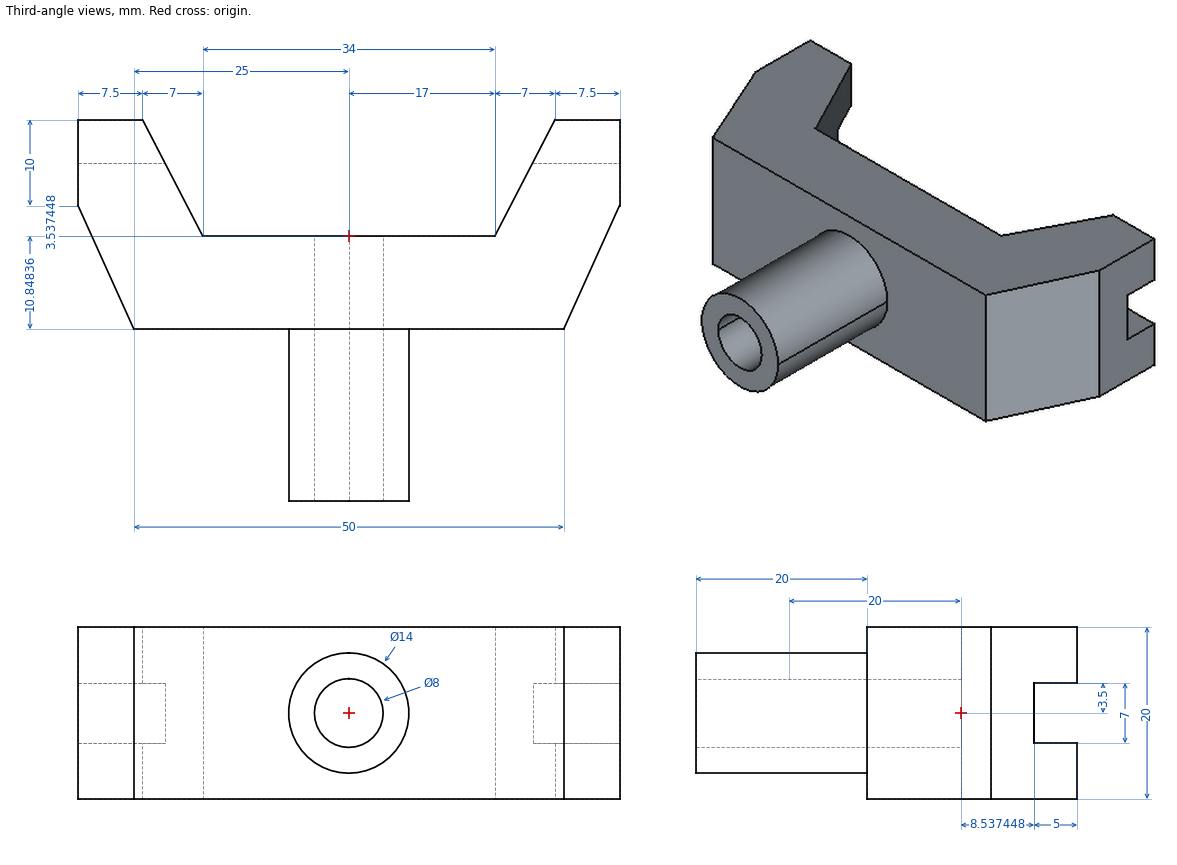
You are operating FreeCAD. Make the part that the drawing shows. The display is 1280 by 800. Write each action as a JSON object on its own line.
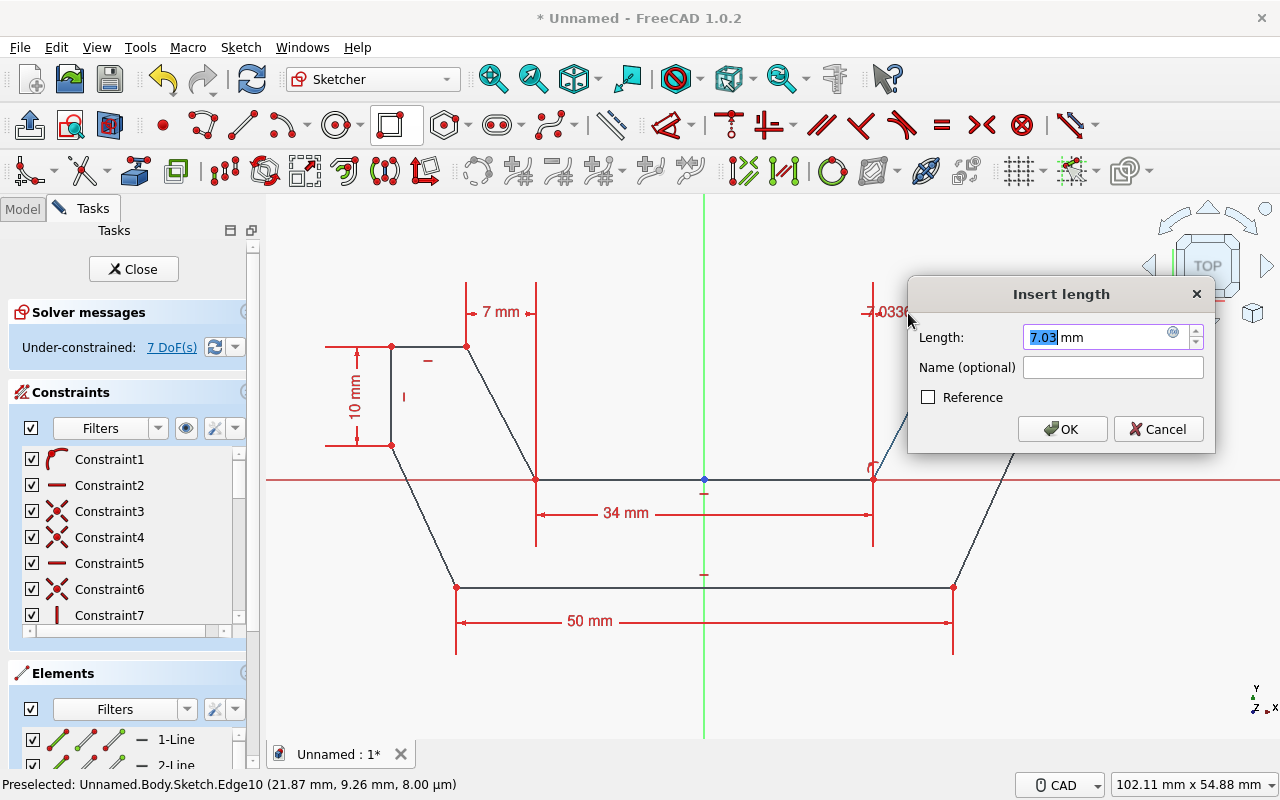
{"action": "type", "text": "7"}
{"action": "key", "text": "Return"}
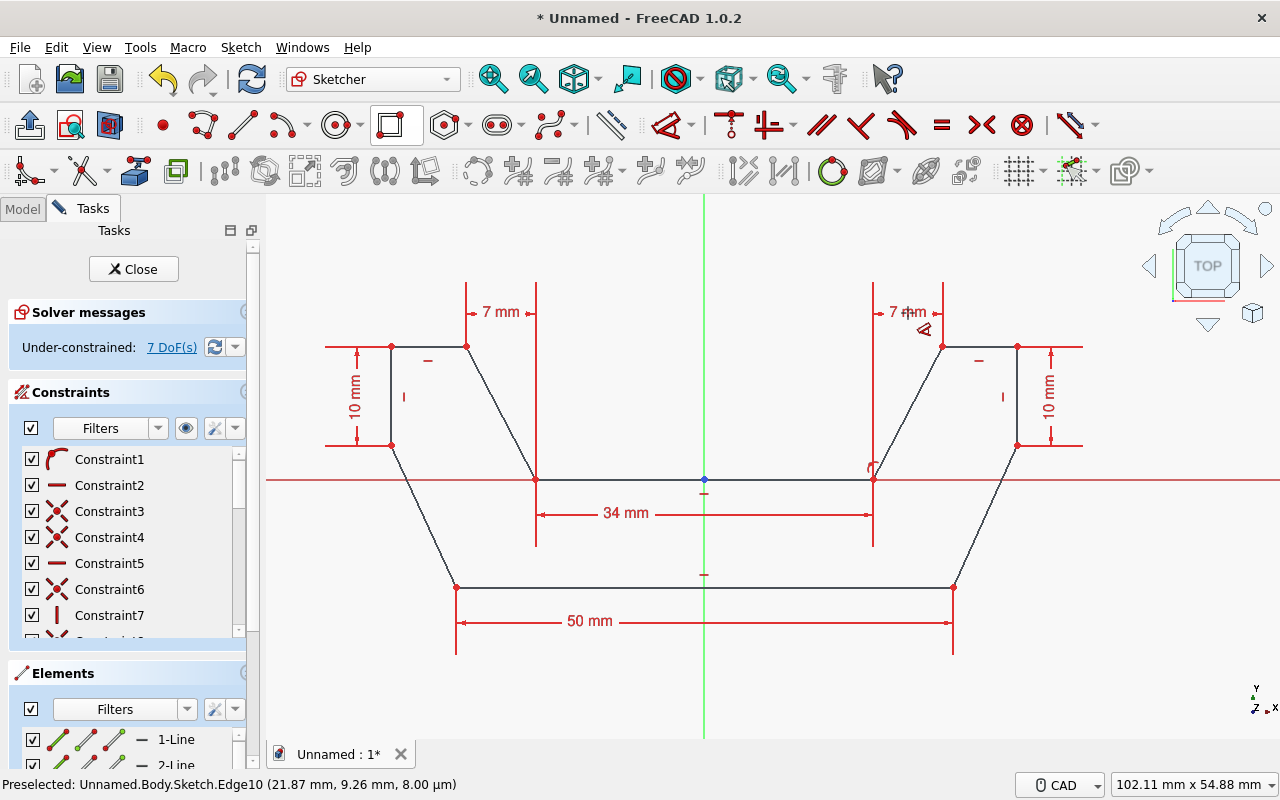
{"action": "left_click", "coordinate": [443, 347]}
{"action": "left_click", "coordinate": [428, 313]}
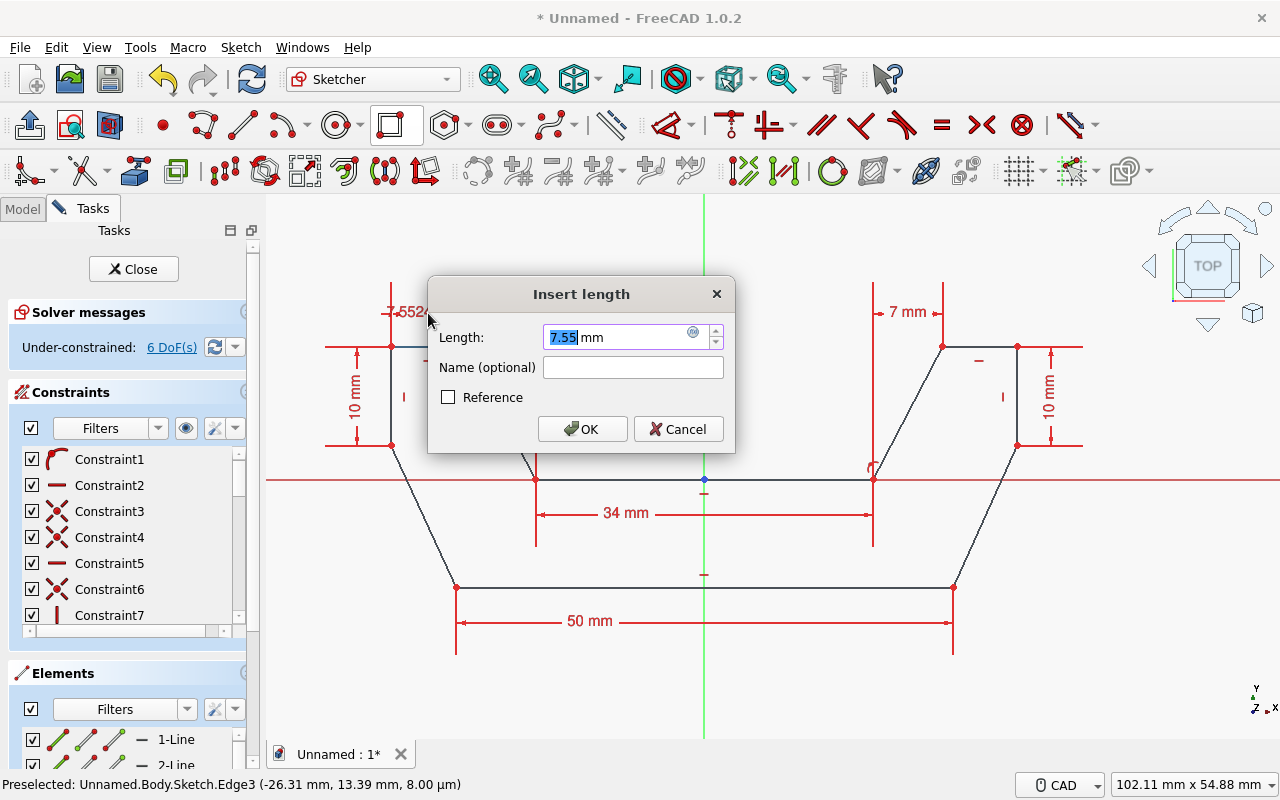
{"action": "type", "text": "7.5"}
{"action": "key", "text": "Return"}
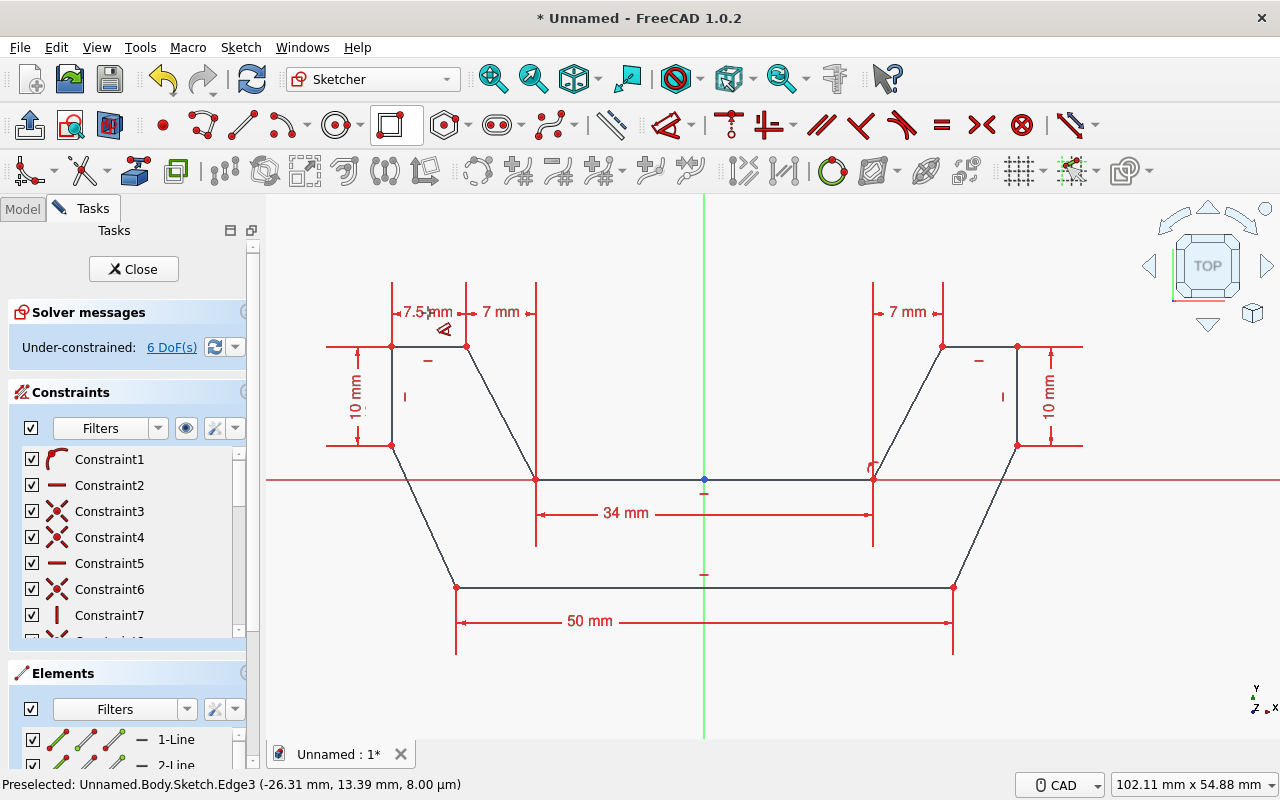
{"action": "left_click", "coordinate": [995, 347]}
{"action": "left_click", "coordinate": [980, 313]}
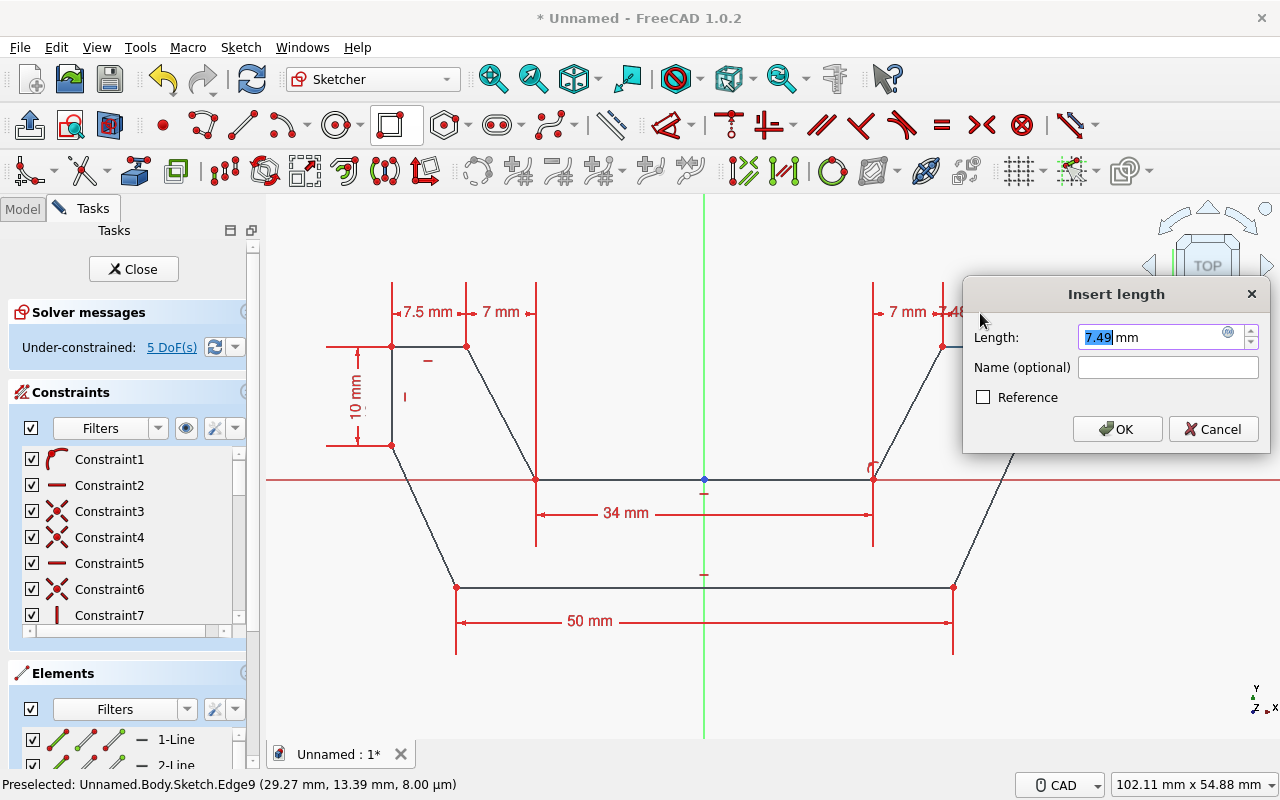
{"action": "type", "text": "7.5"}
{"action": "key", "text": "Return"}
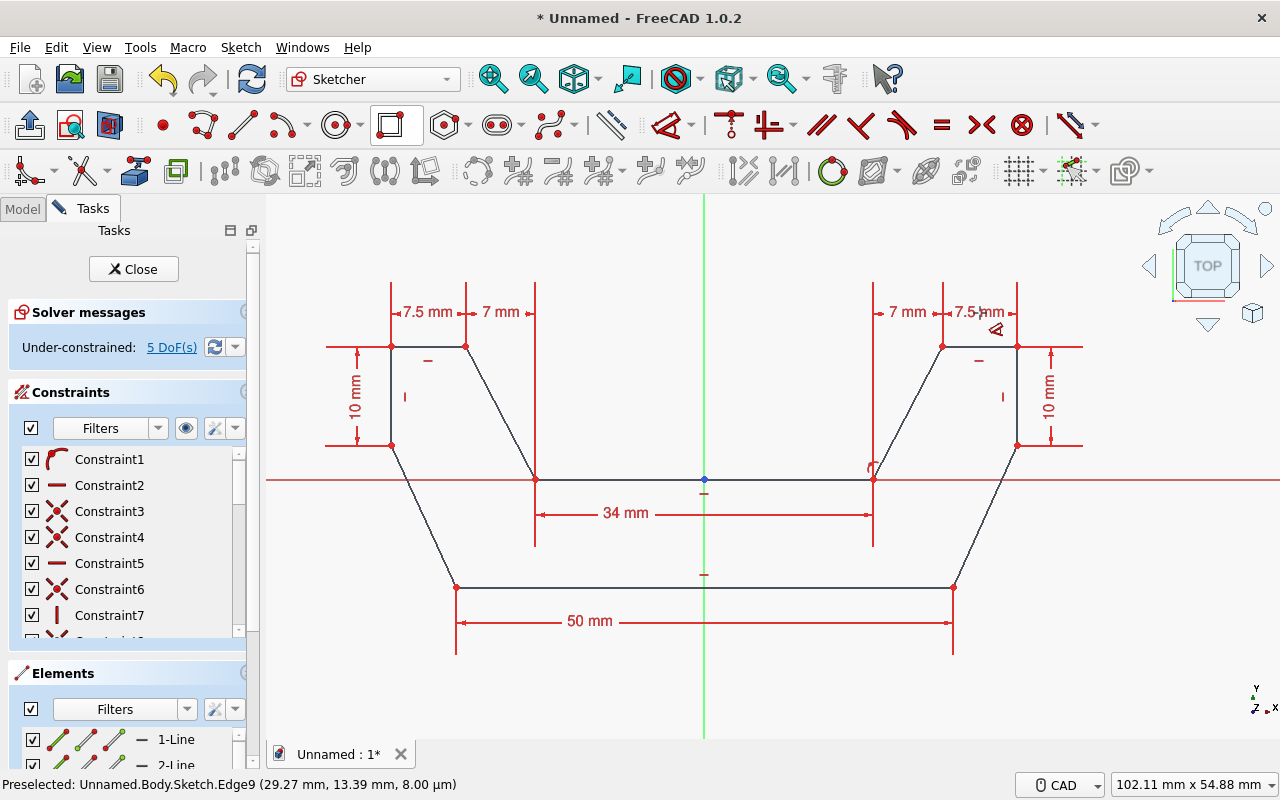
{"action": "left_click", "coordinate": [873, 480]}
{"action": "left_click", "coordinate": [789, 514]}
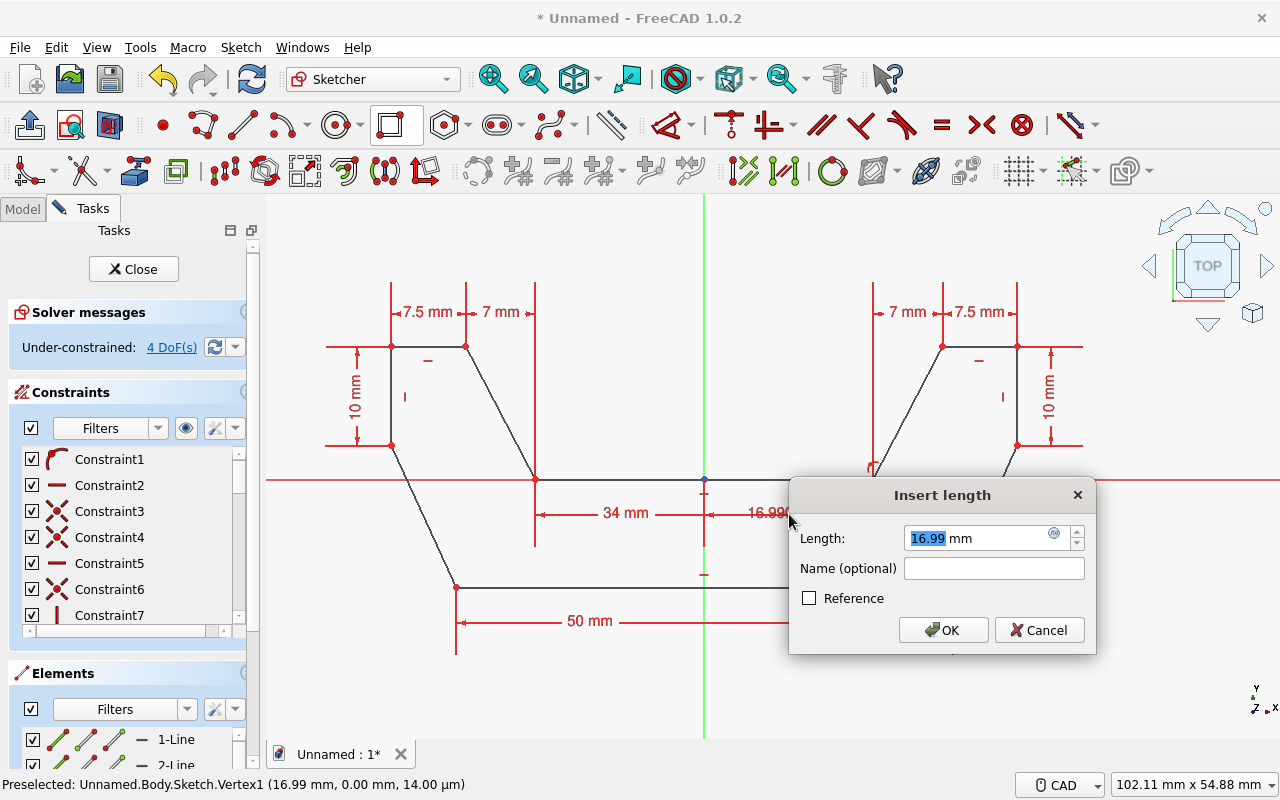
{"action": "type", "text": "17"}
{"action": "key", "text": "Return"}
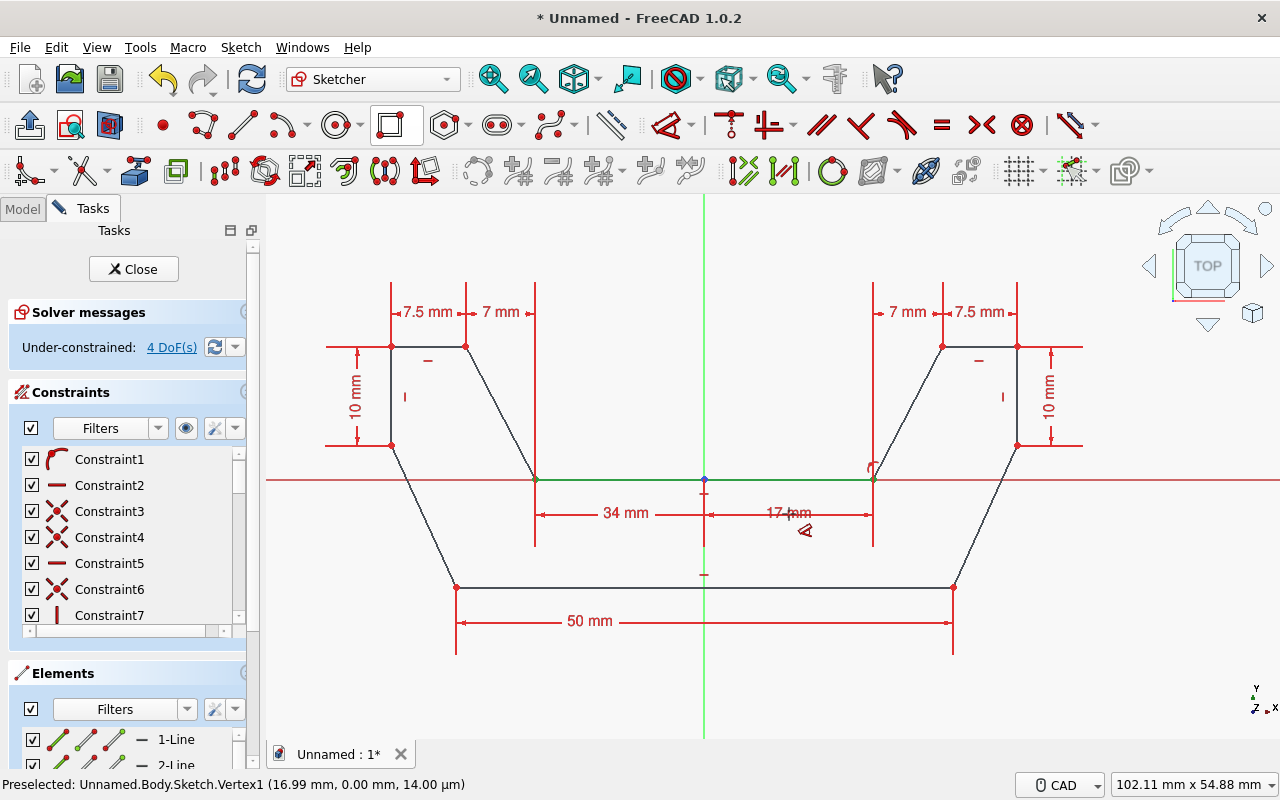
{"action": "left_click", "coordinate": [456, 588]}
{"action": "left_click", "coordinate": [494, 622]}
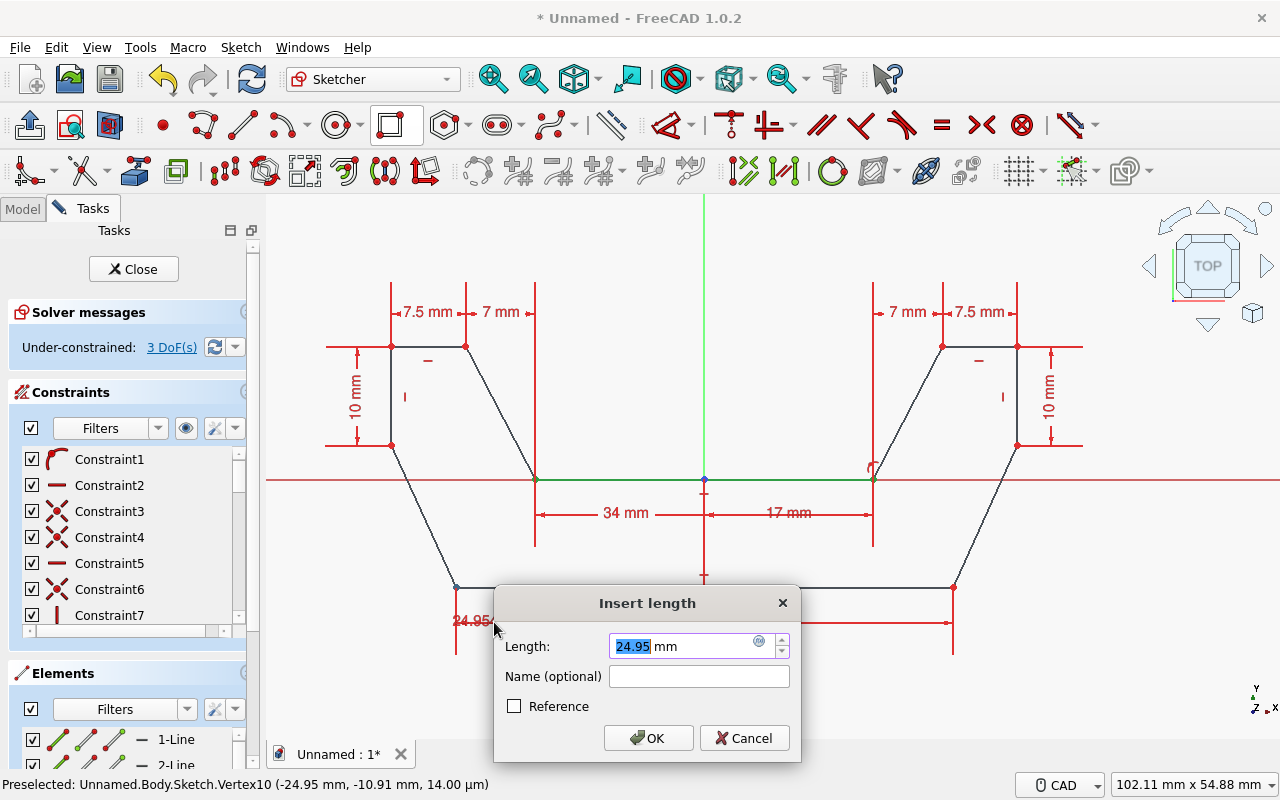
{"action": "type", "text": "25"}
{"action": "key", "text": "Return"}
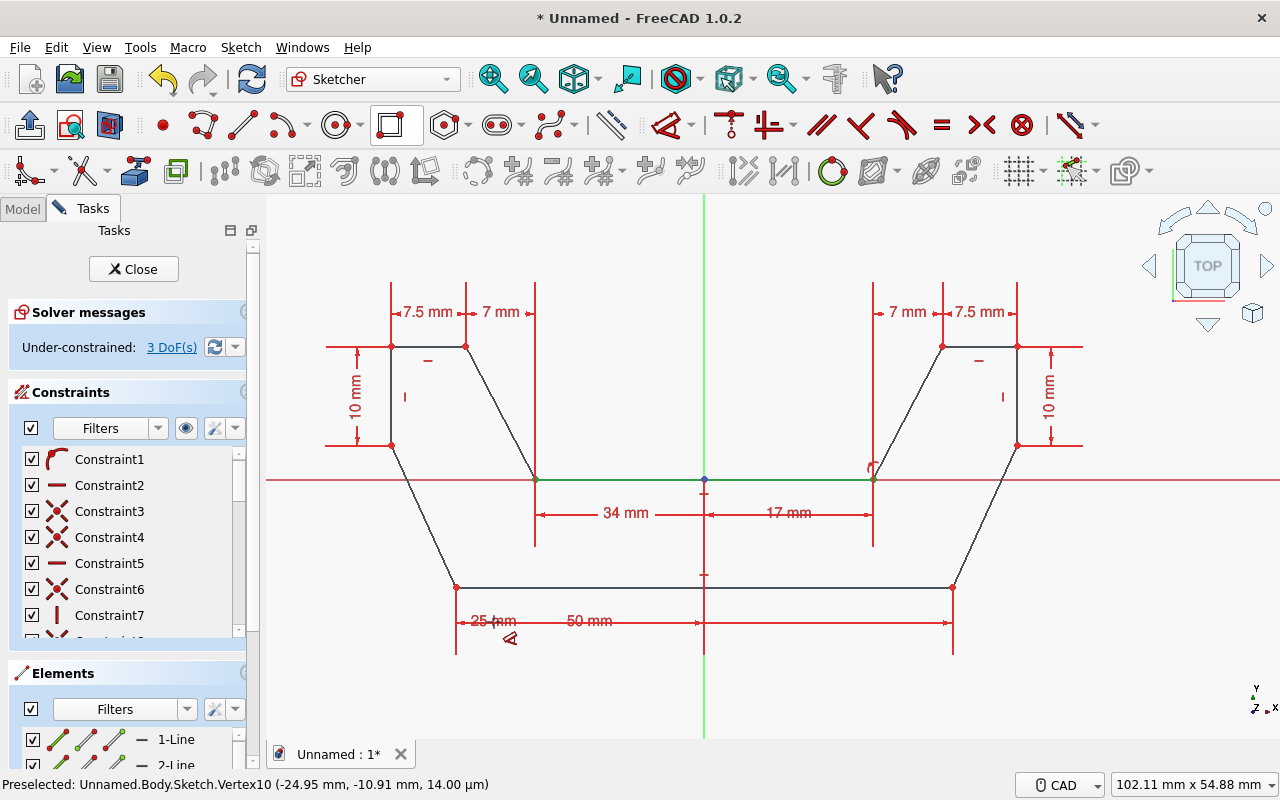
{"action": "left_click", "coordinate": [391, 446]}
{"action": "left_click", "coordinate": [357, 463]}